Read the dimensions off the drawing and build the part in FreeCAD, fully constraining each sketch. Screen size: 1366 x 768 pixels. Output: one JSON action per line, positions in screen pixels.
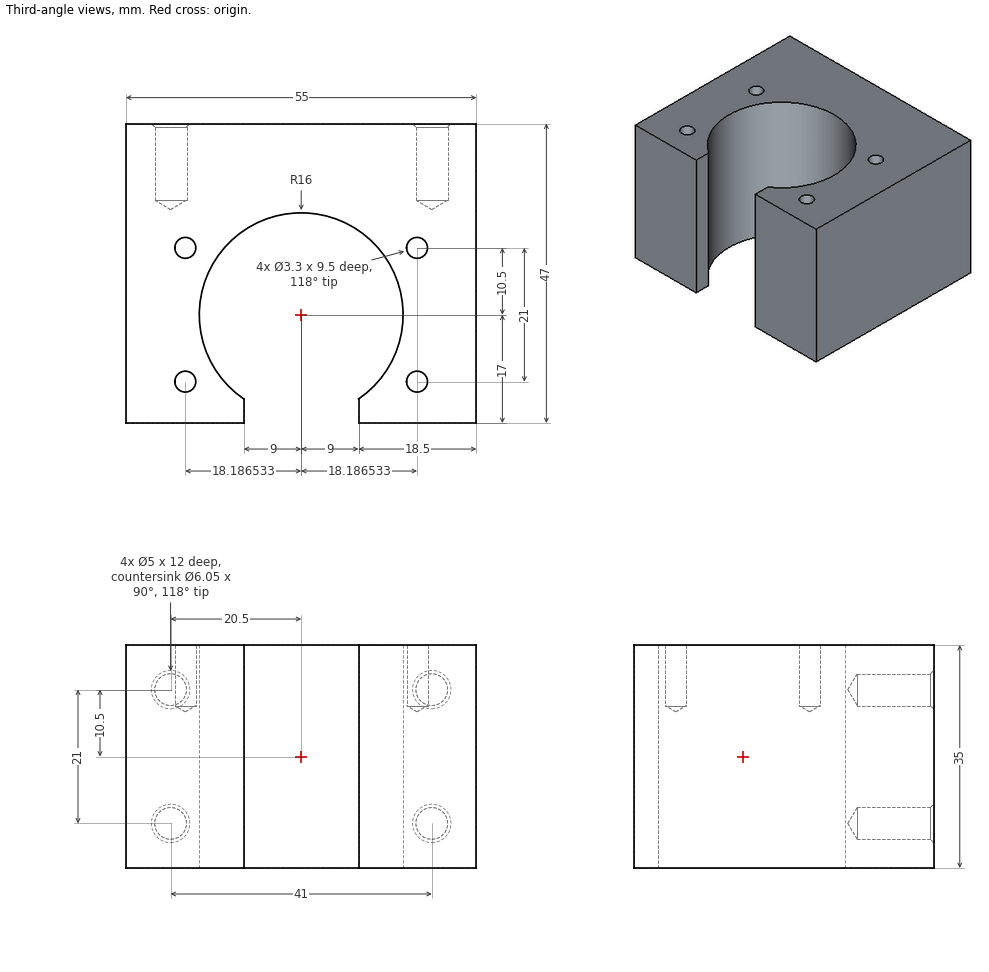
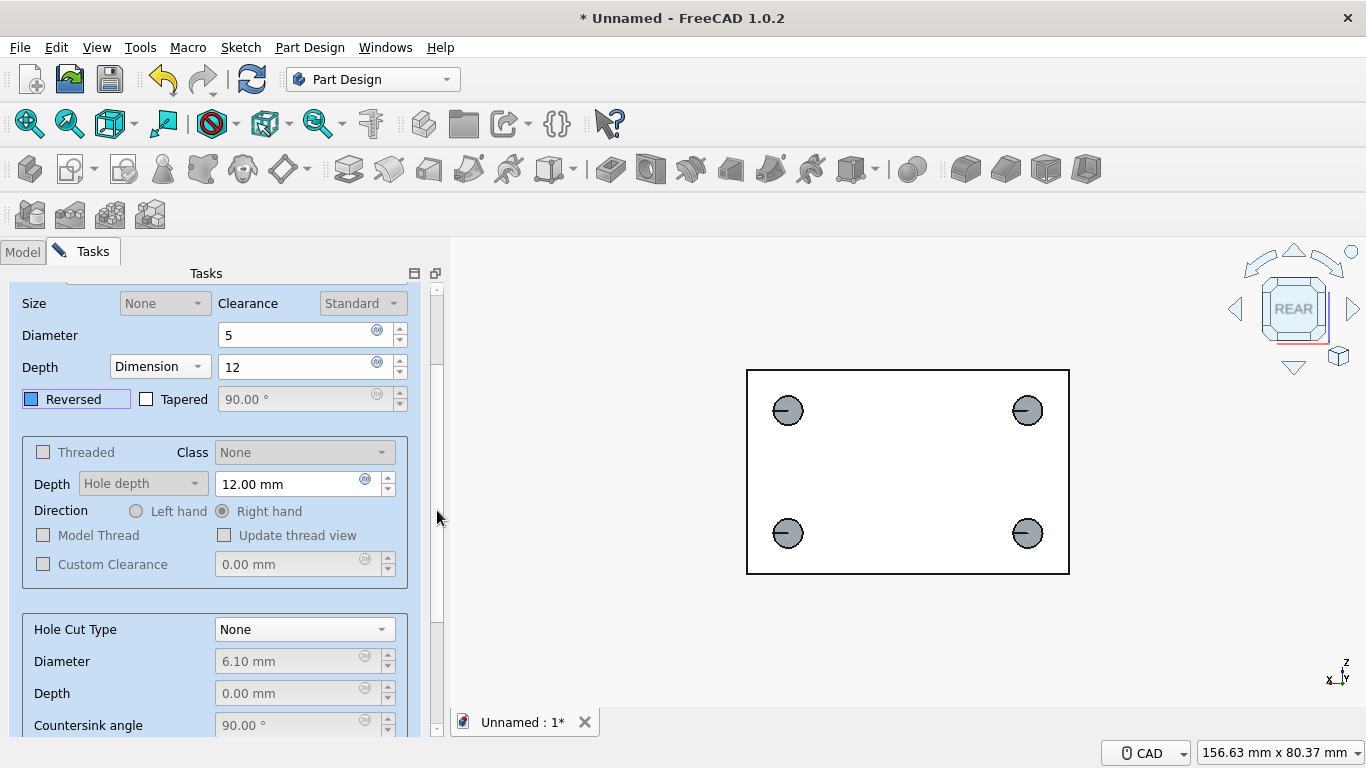
{"action": "left_click", "coordinate": [306, 630]}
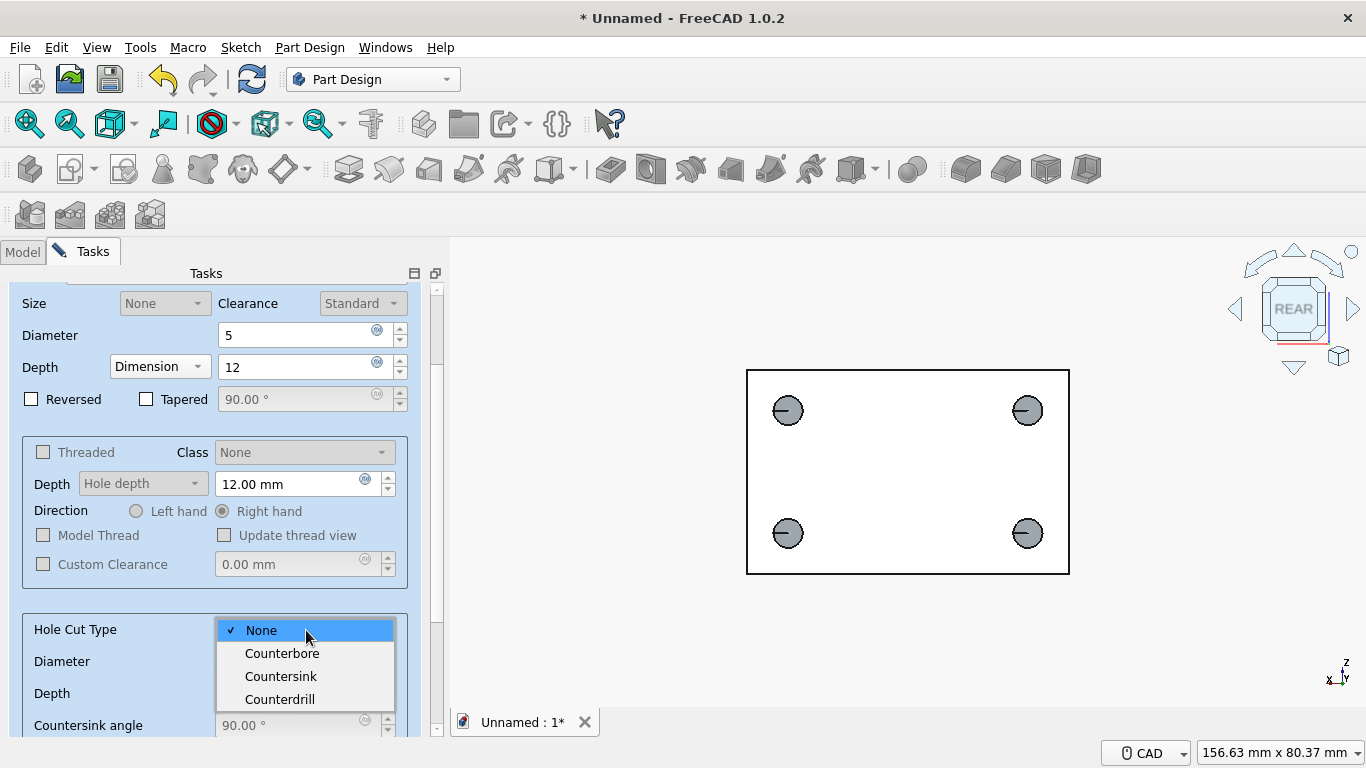
{"action": "left_click", "coordinate": [304, 676]}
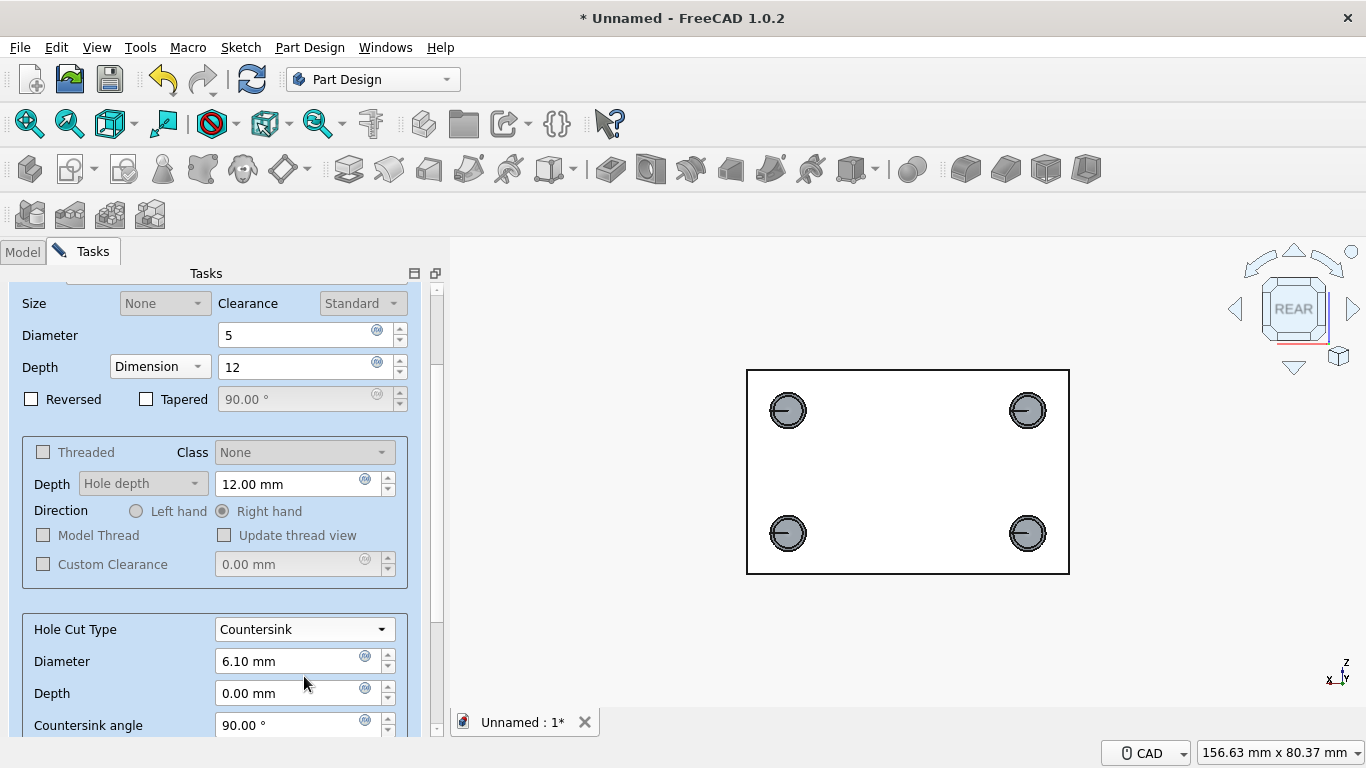
{"action": "triple_click", "coordinate": [298, 661]}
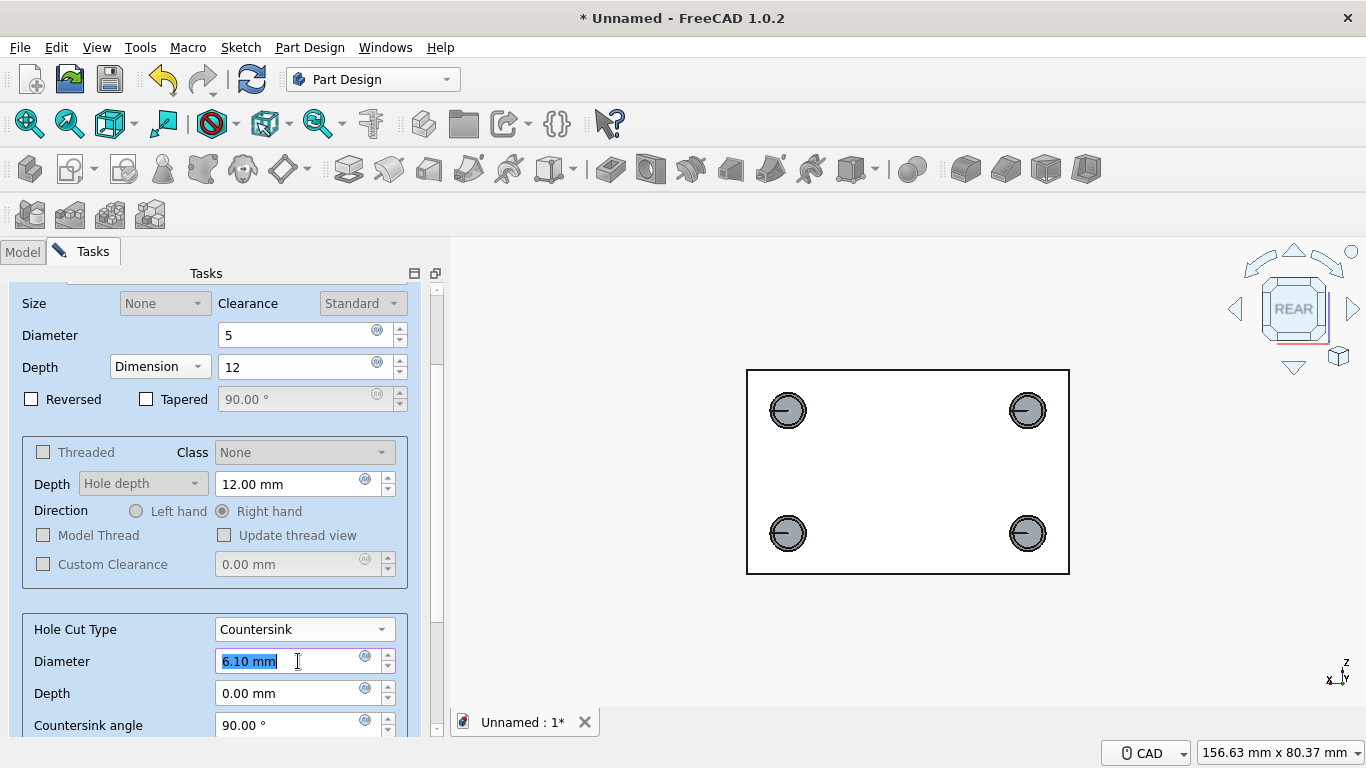
{"action": "type", "text": "6.05"}
{"action": "key", "text": "Tab"}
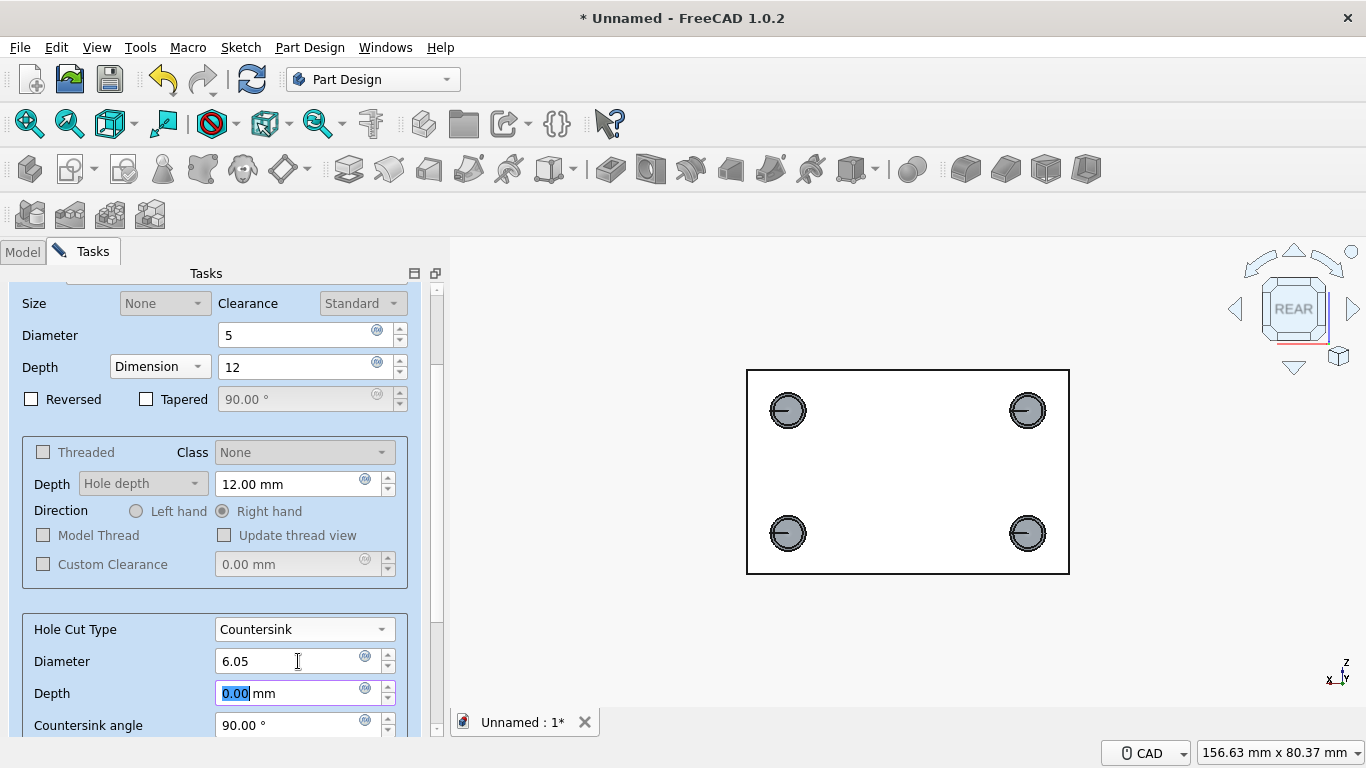
{"action": "scroll", "coordinate": [437, 510], "scroll_direction": "up", "scroll_amount": 3}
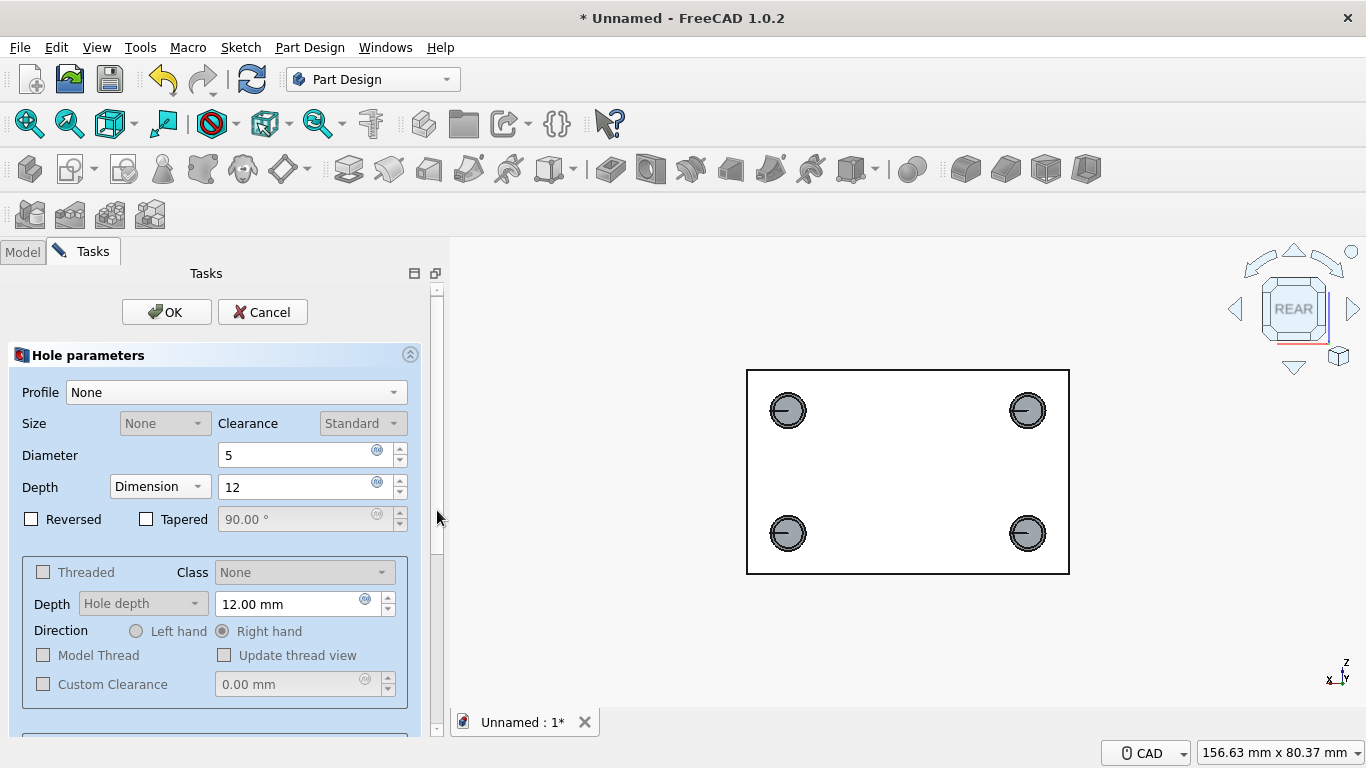
{"action": "left_click", "coordinate": [167, 312]}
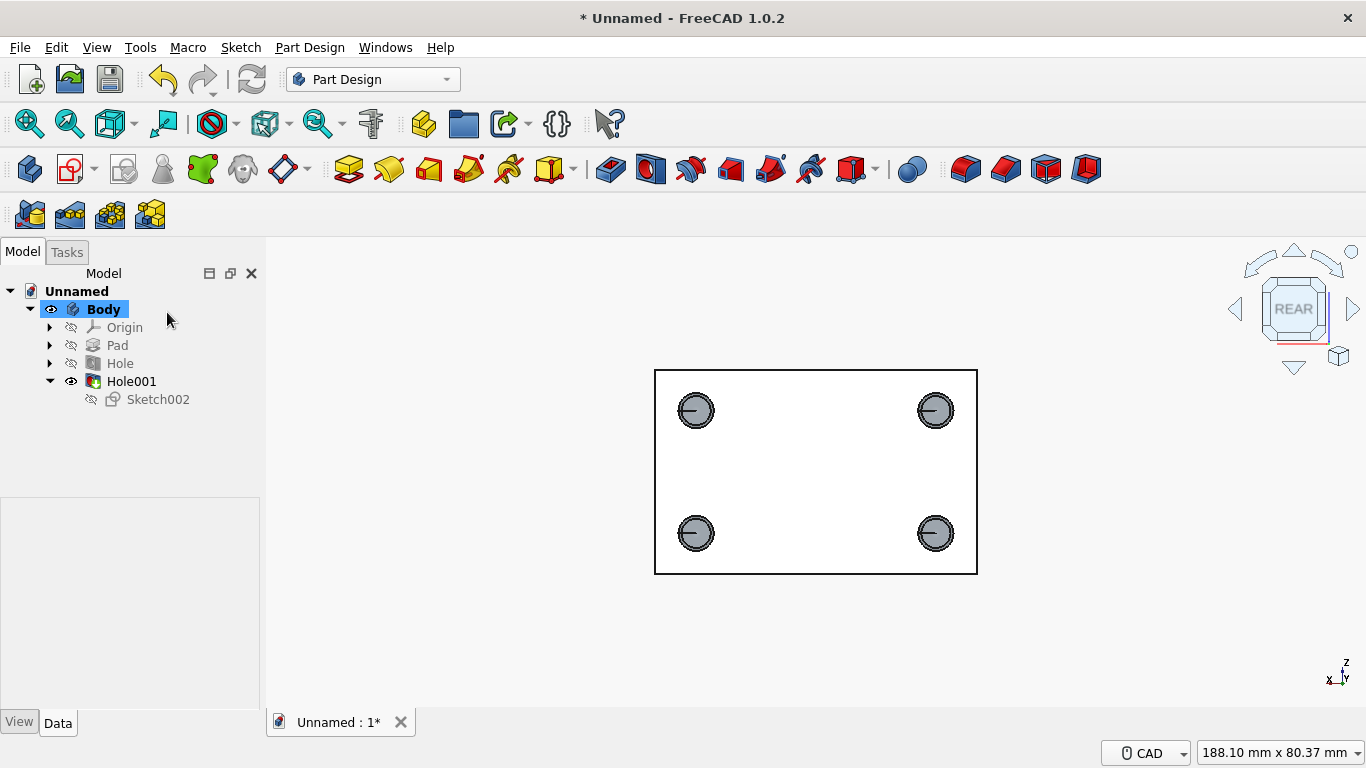
{"action": "key", "text": "0"}